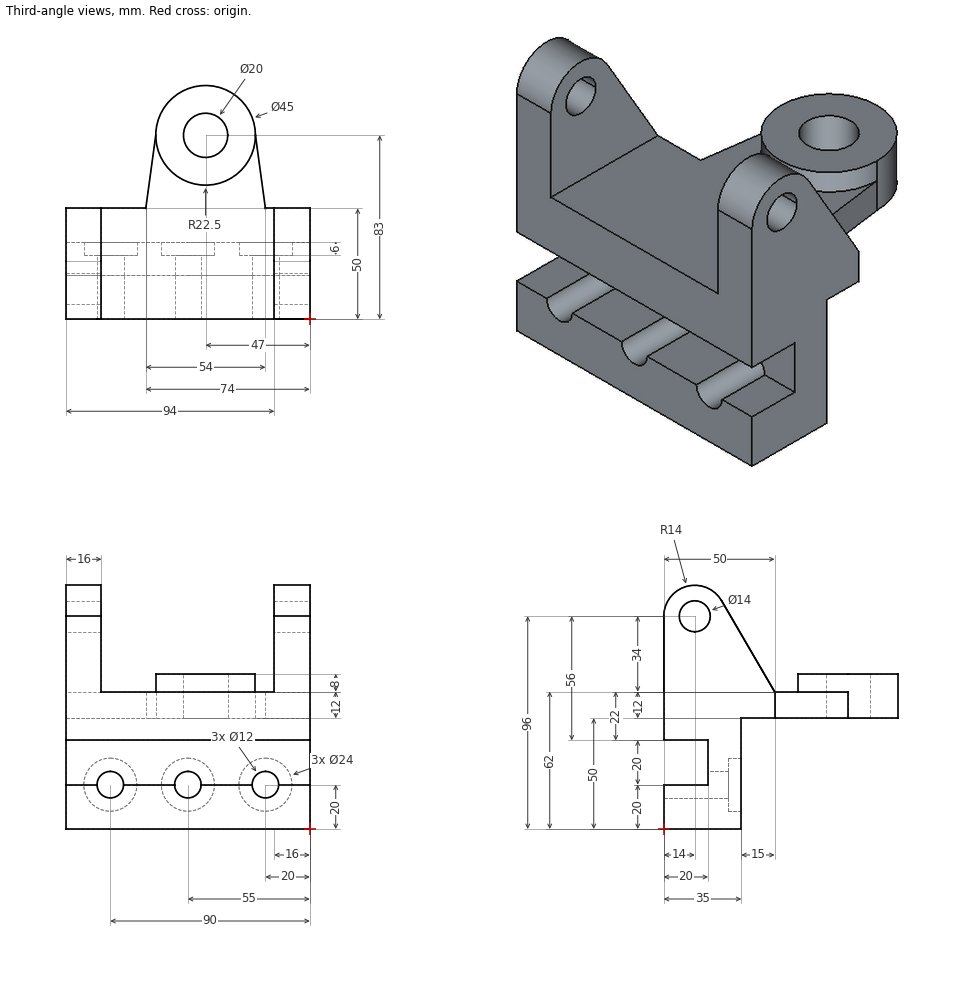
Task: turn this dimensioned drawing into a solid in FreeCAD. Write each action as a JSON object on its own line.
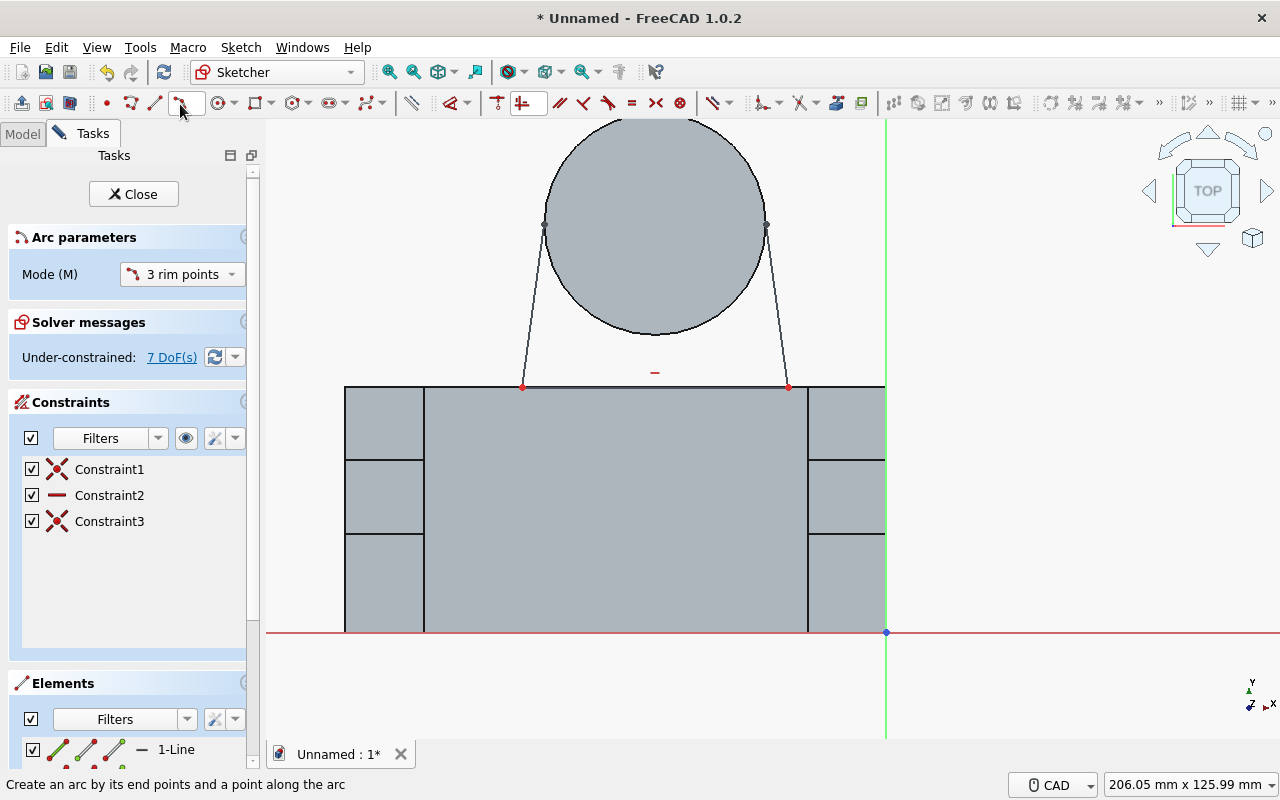
{"action": "left_click", "coordinate": [766, 225]}
{"action": "left_click", "coordinate": [544, 225]}
{"action": "left_click", "coordinate": [655, 335]}
{"action": "key", "text": "Escape"}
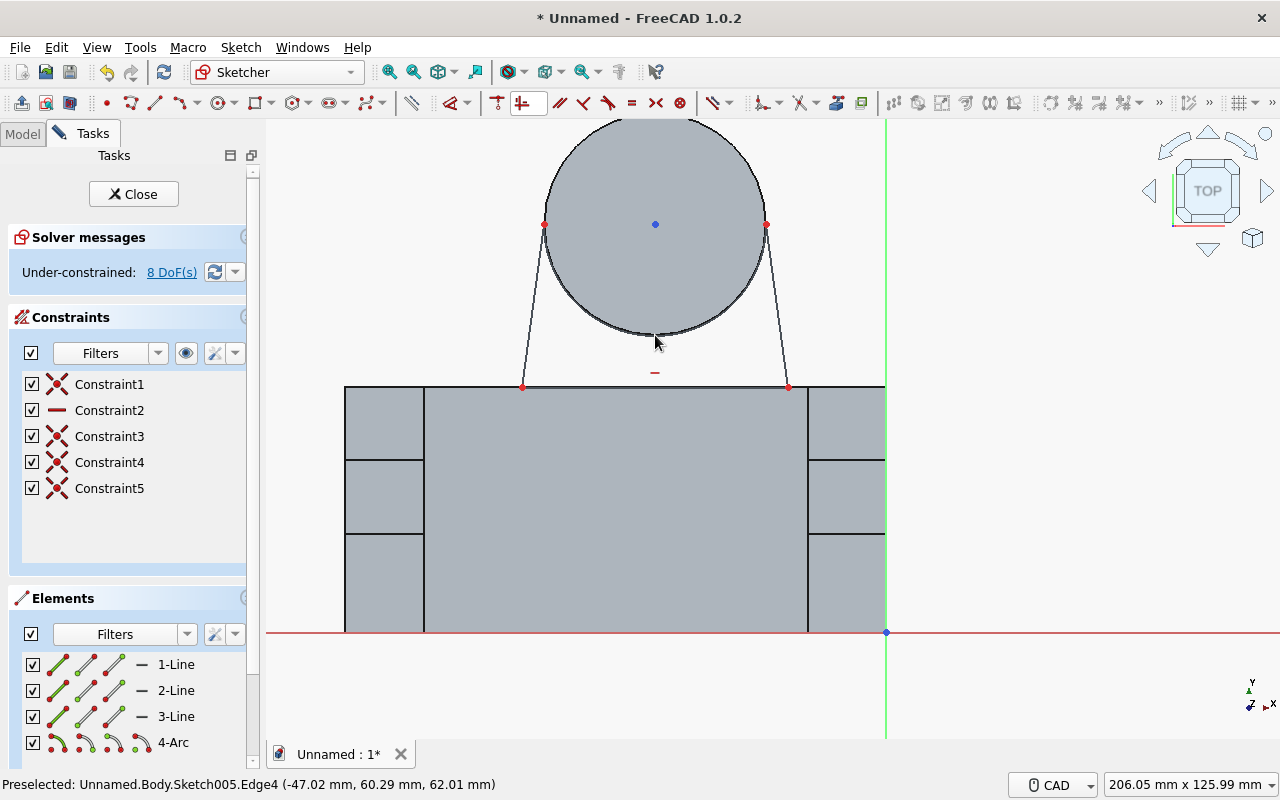
{"action": "key", "text": "d"}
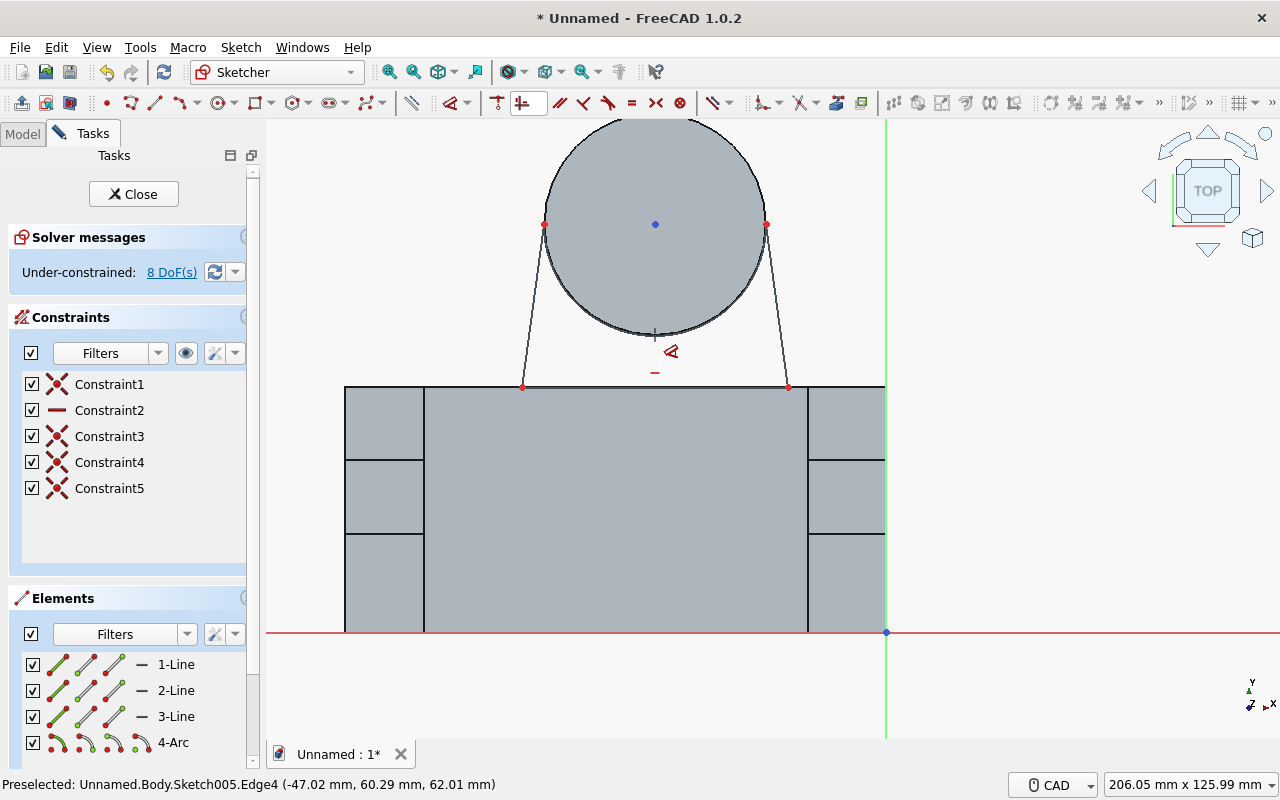
{"action": "left_click", "coordinate": [590, 315]}
{"action": "left_click", "coordinate": [571, 341]}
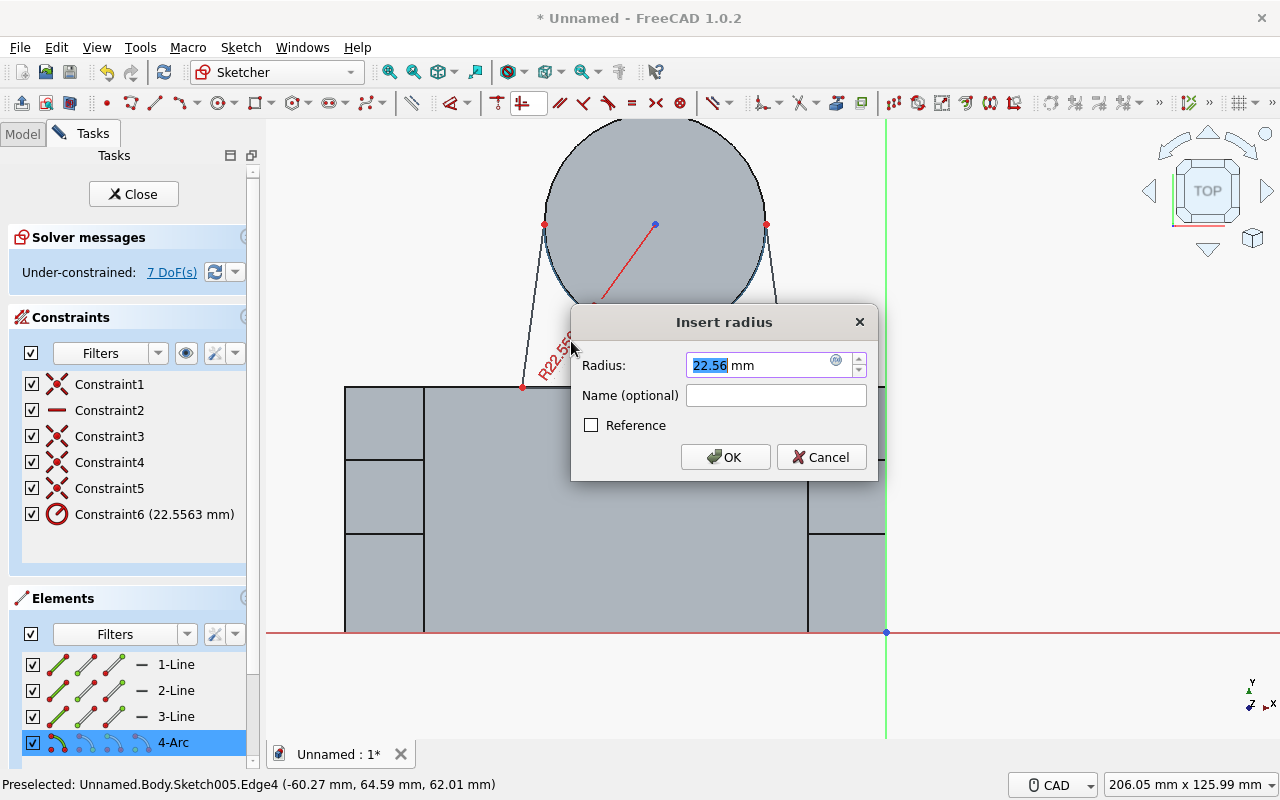
{"action": "type", "text": "22.5"}
{"action": "key", "text": "Return"}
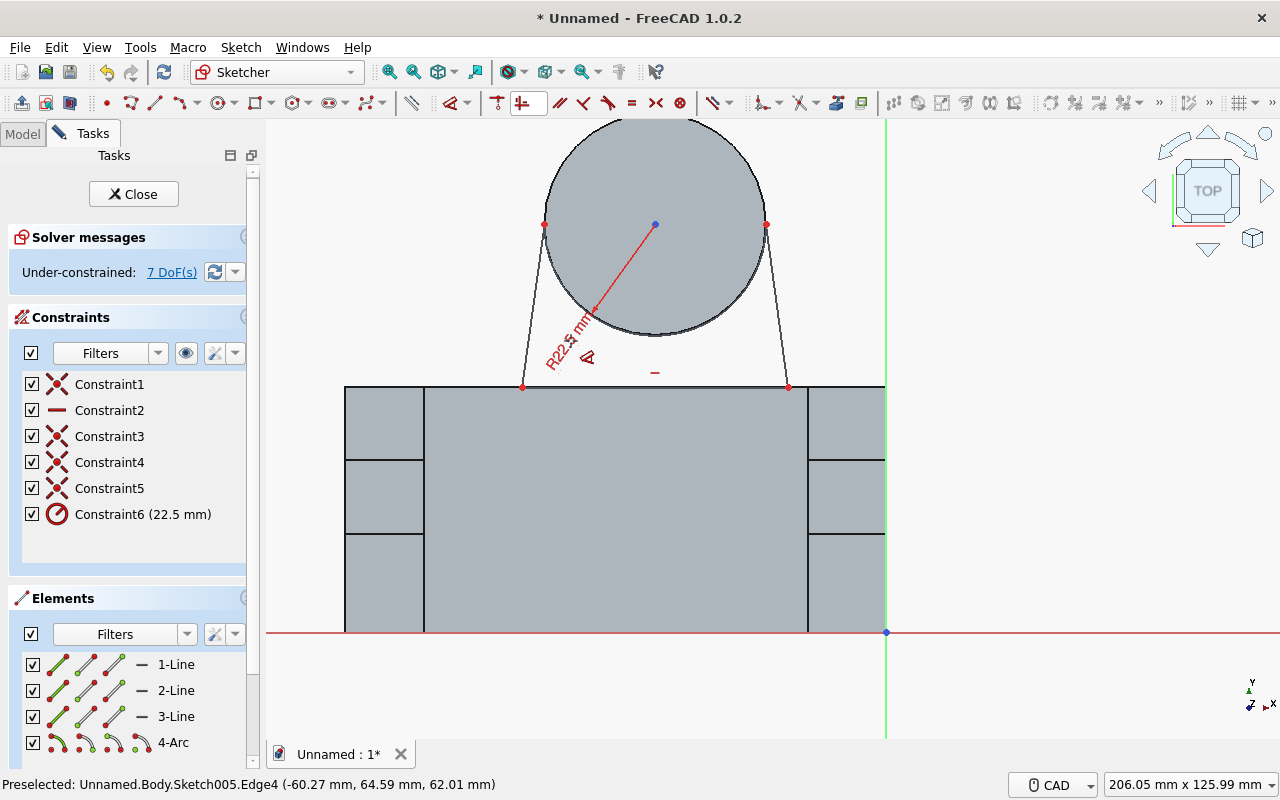
{"action": "left_click", "coordinate": [602, 388]}
{"action": "left_click", "coordinate": [655, 354]}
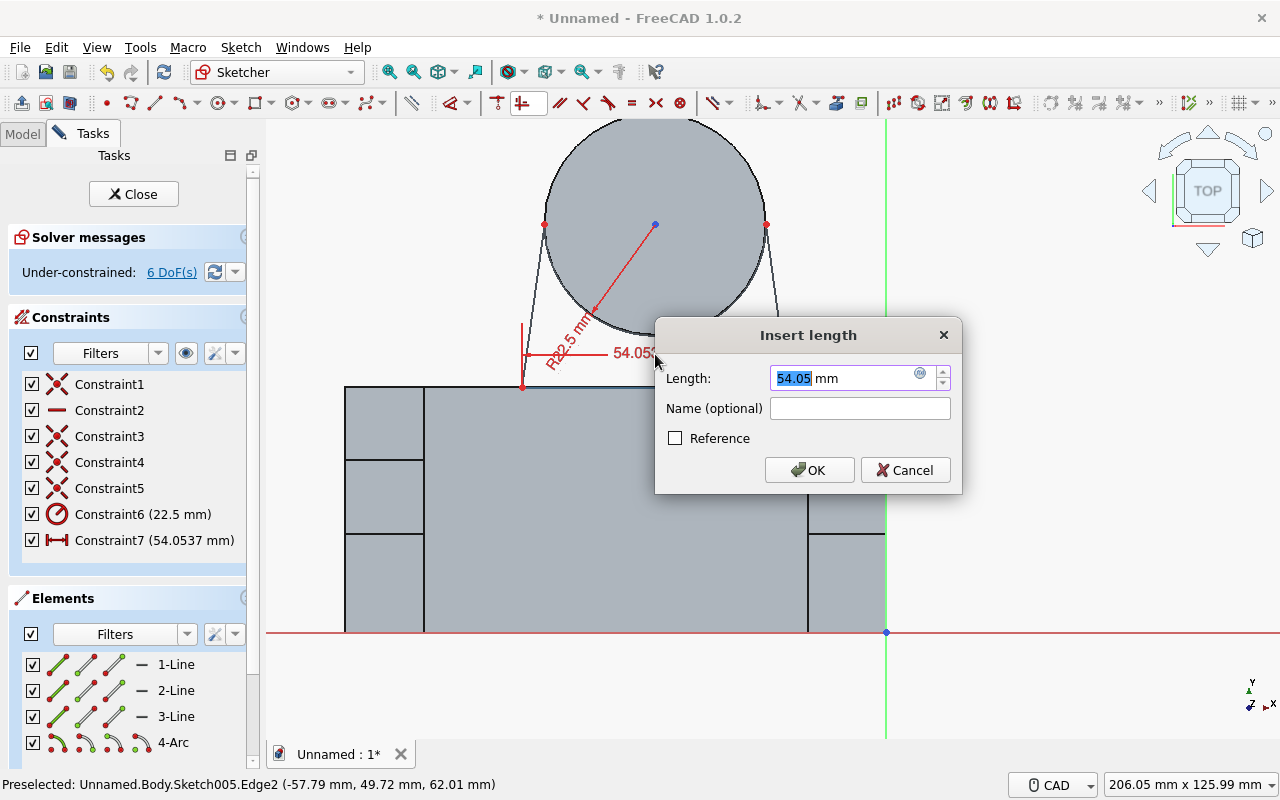
{"action": "type", "text": "54"}
{"action": "key", "text": "Return"}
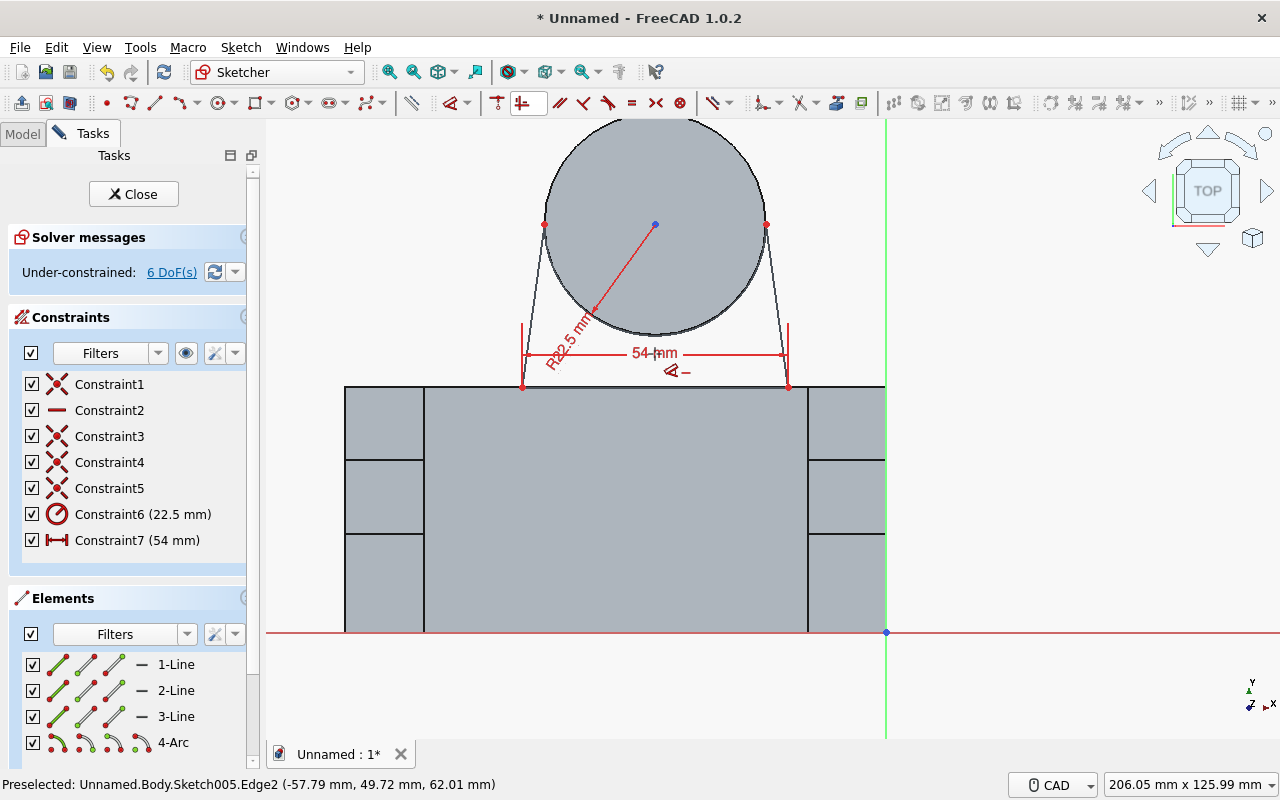
{"action": "left_click", "coordinate": [545, 225]}
{"action": "left_click", "coordinate": [920, 429]}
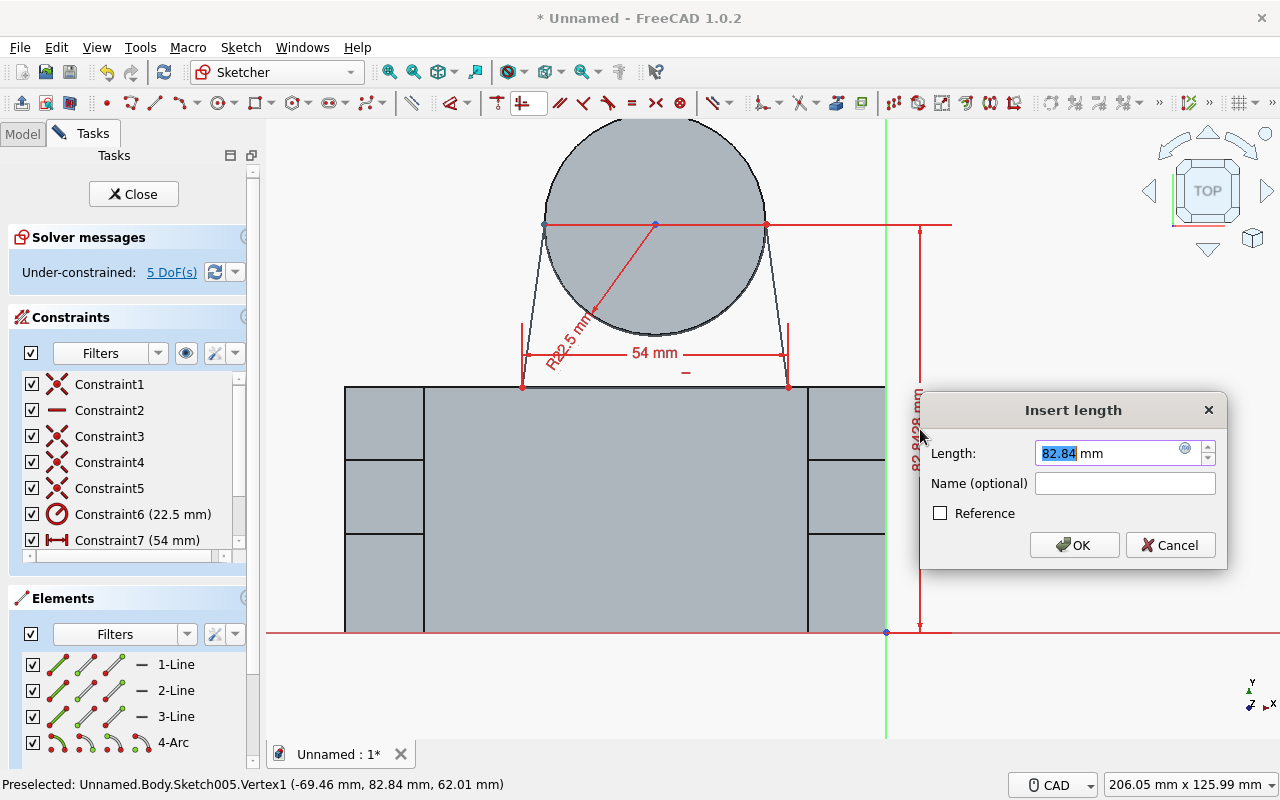
{"action": "type", "text": "83"}
{"action": "key", "text": "Return"}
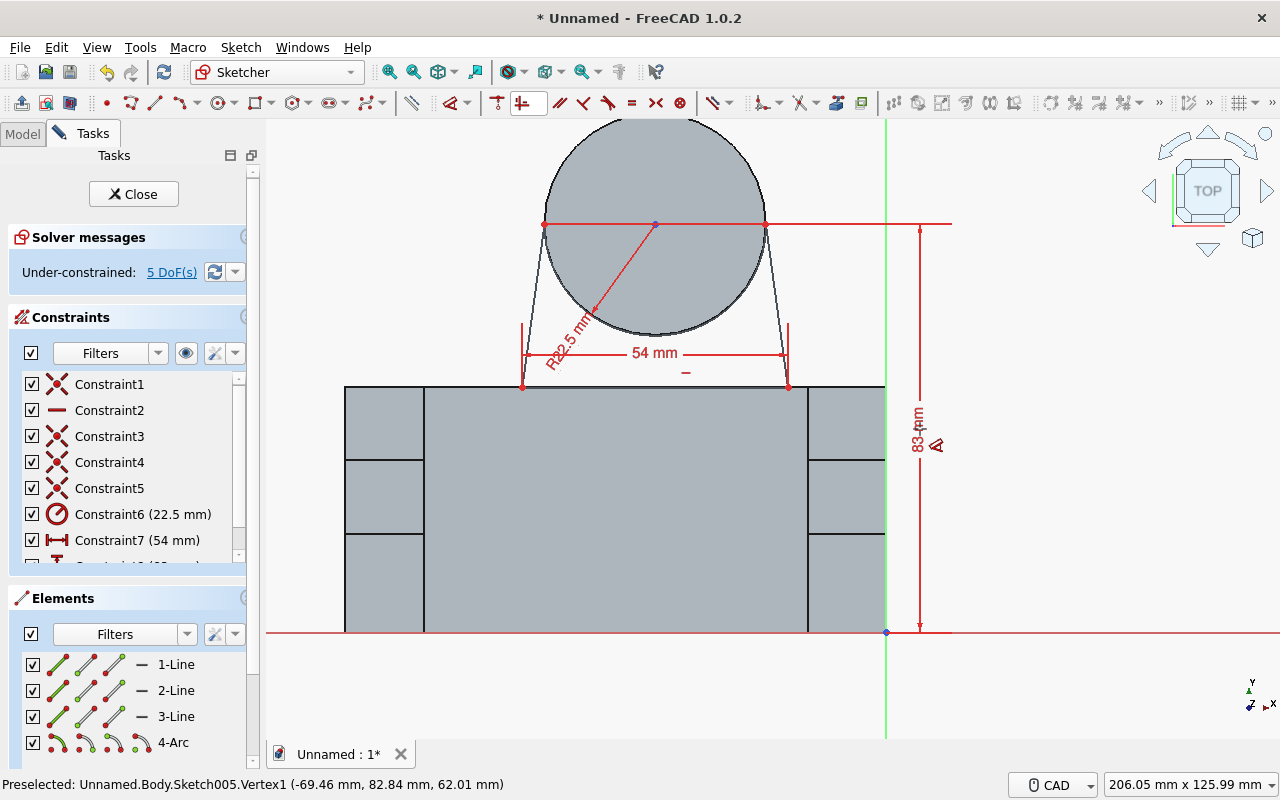
{"action": "left_click", "coordinate": [522, 388]}
{"action": "left_click", "coordinate": [704, 667]}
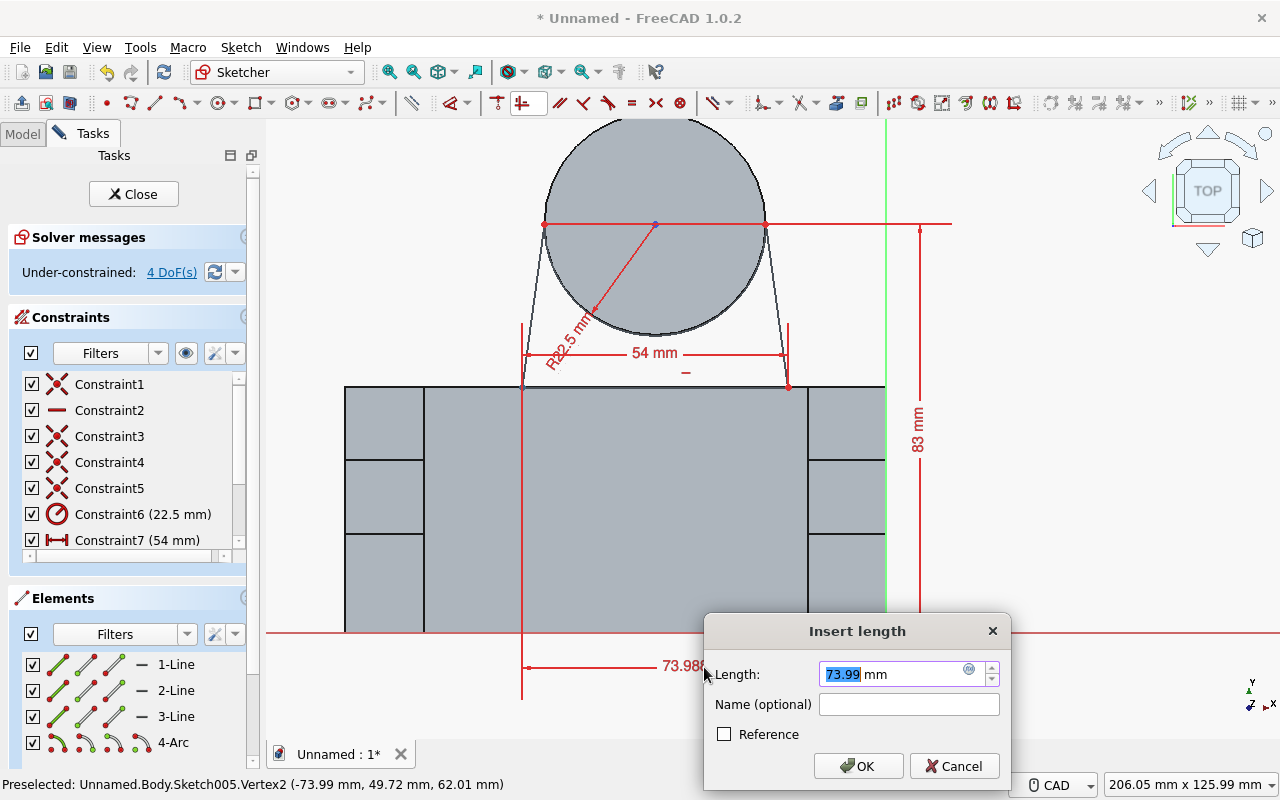
{"action": "type", "text": "74"}
{"action": "key", "text": "Return"}